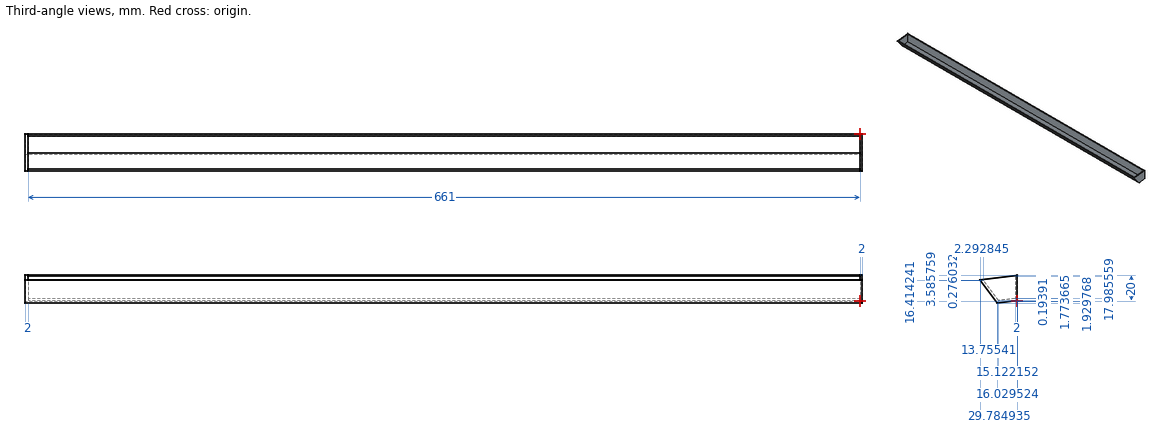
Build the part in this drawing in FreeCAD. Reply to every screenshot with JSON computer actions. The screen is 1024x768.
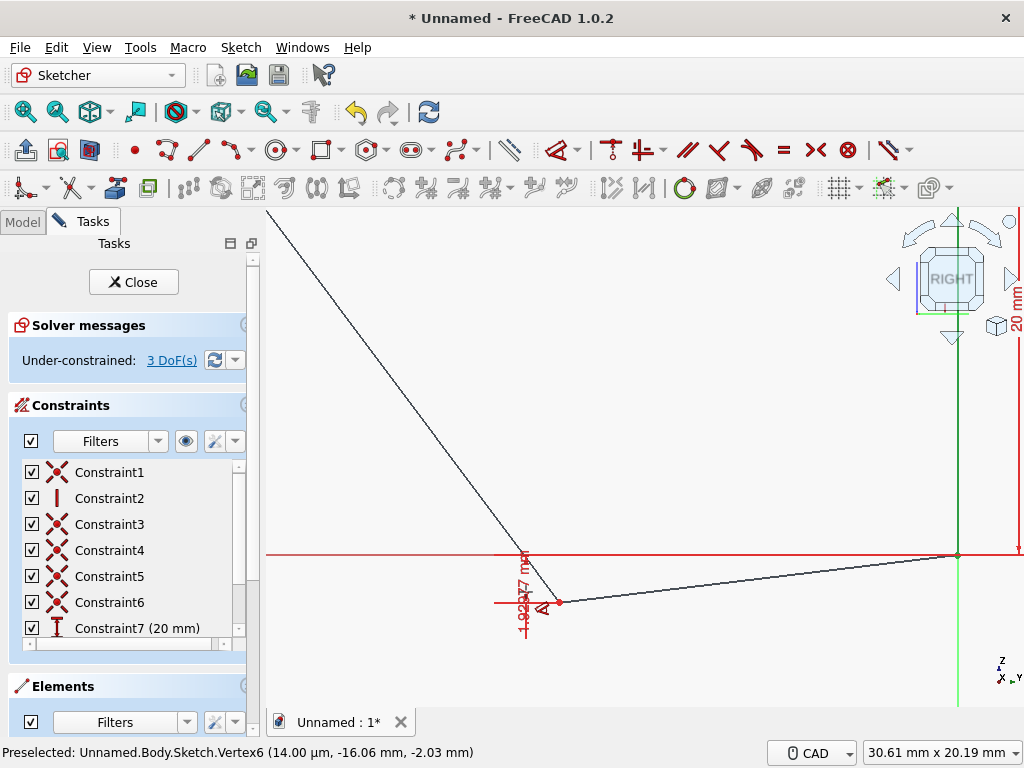
{"action": "scroll", "coordinate": [562, 610], "scroll_direction": "down", "scroll_amount": 3}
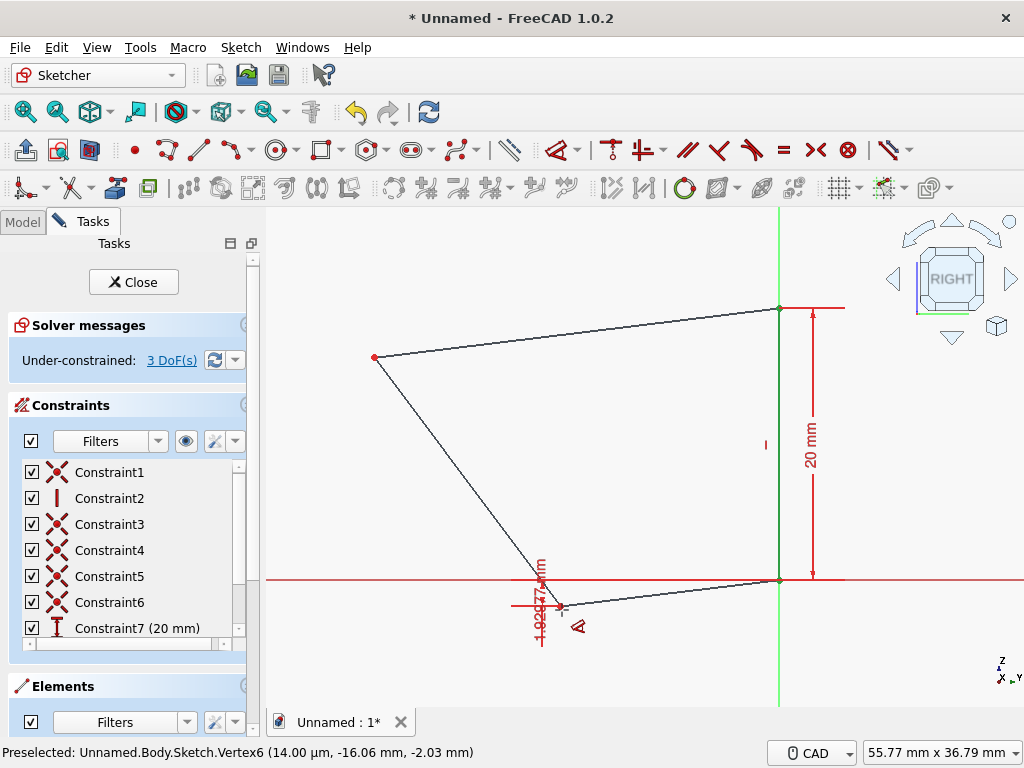
{"action": "left_click", "coordinate": [658, 323]}
{"action": "left_click", "coordinate": [813, 333]}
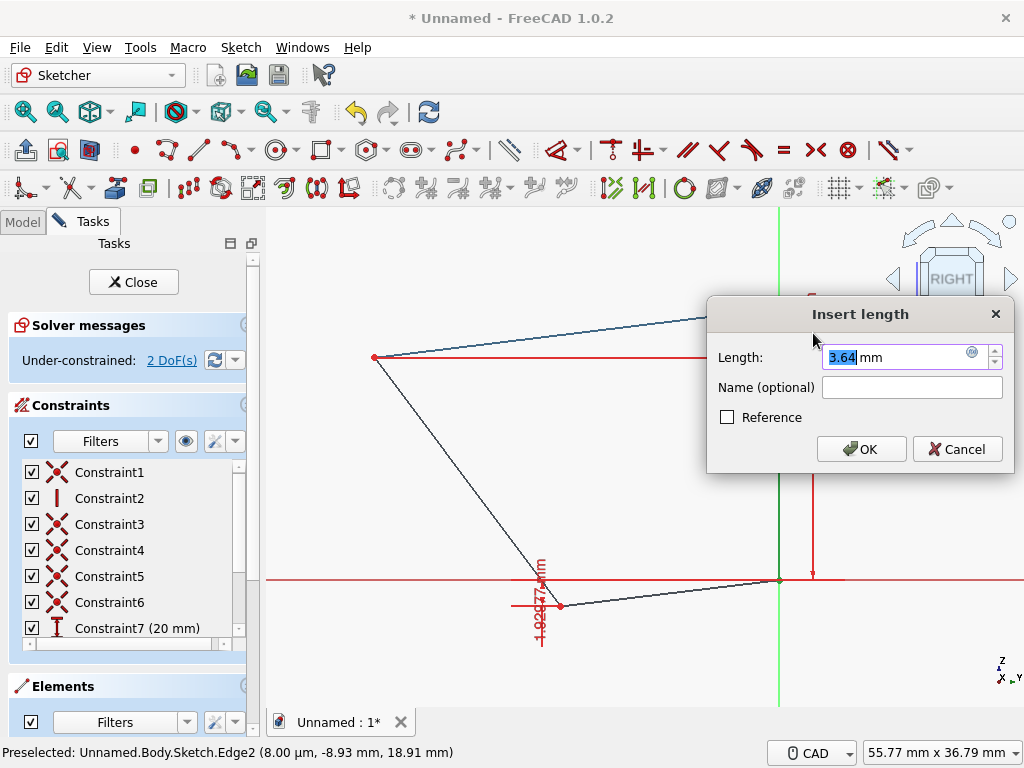
{"action": "type", "text": "3.585759"}
{"action": "key", "text": "Return"}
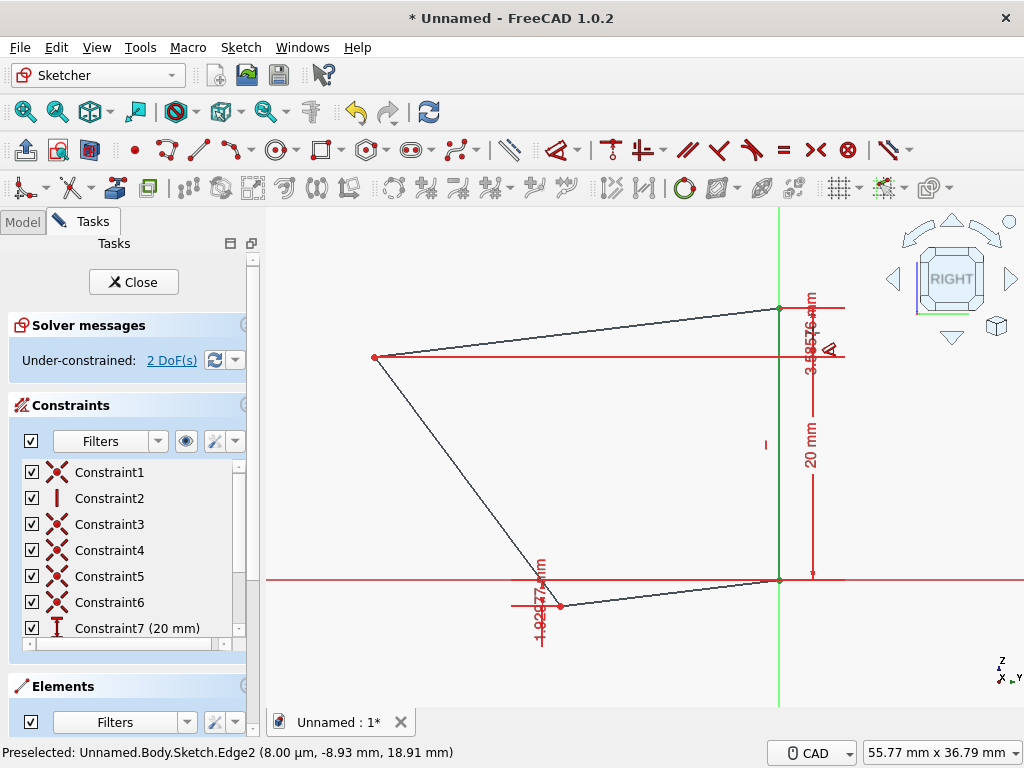
{"action": "left_click", "coordinate": [431, 432]}
{"action": "left_click", "coordinate": [468, 640]}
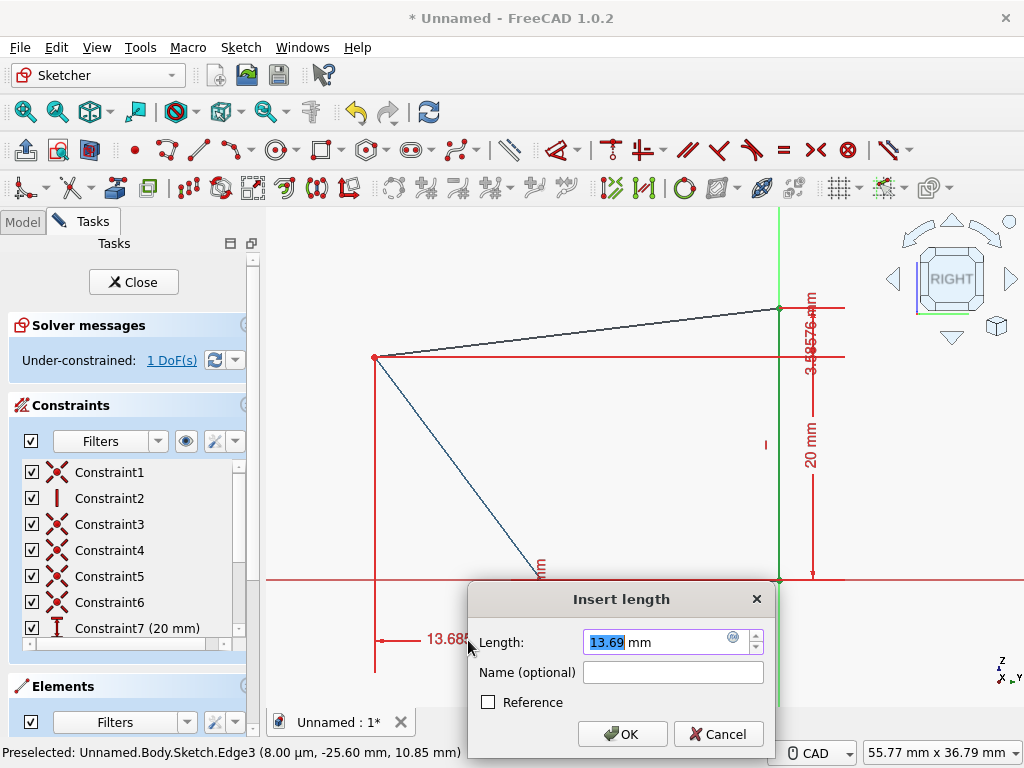
{"action": "type", "text": "13.75541"}
{"action": "key", "text": "Return"}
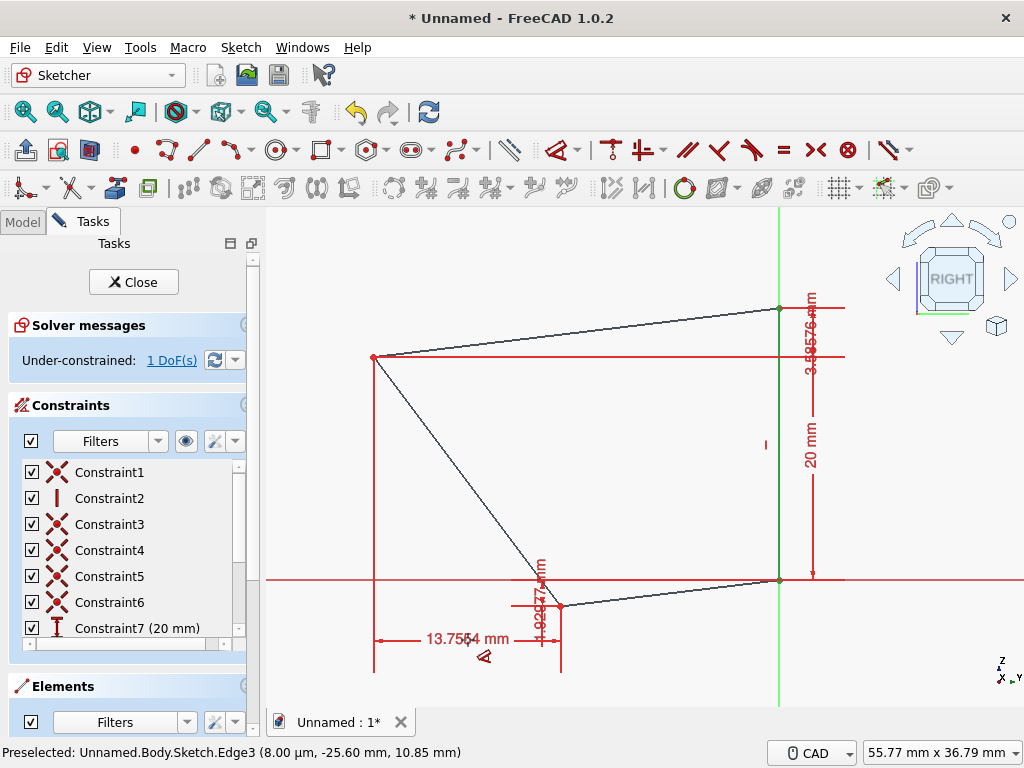
{"action": "left_click", "coordinate": [374, 357]}
{"action": "left_click", "coordinate": [670, 614]}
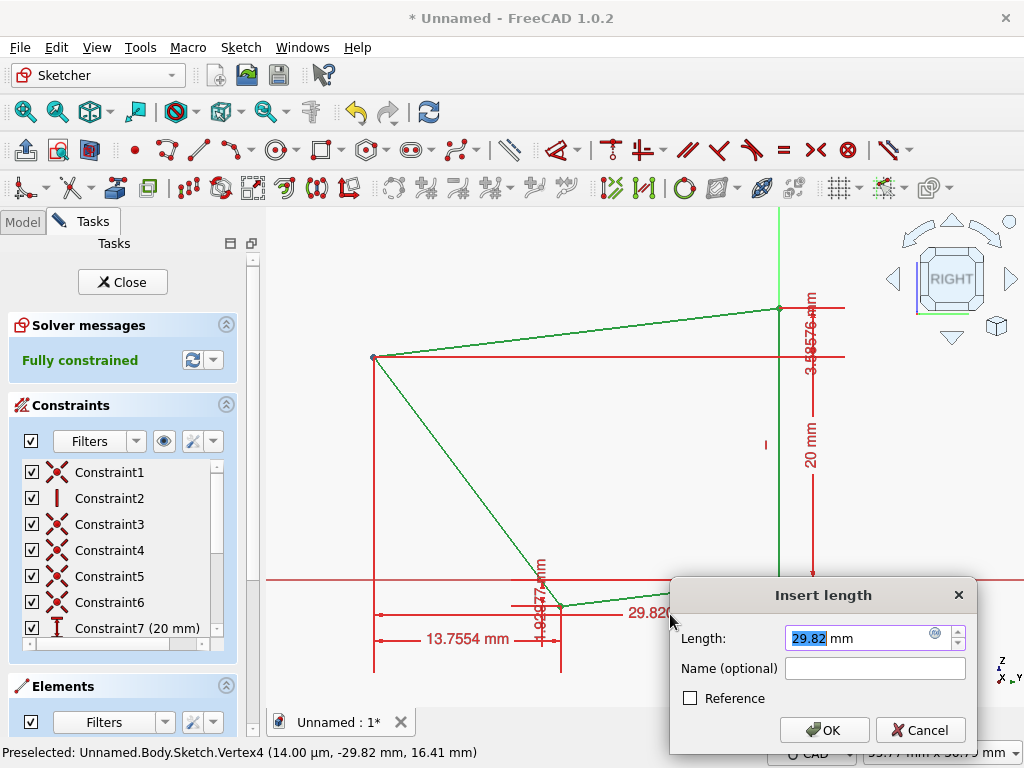
{"action": "type", "text": "29.784935"}
{"action": "key", "text": "Return"}
{"action": "key", "text": "Escape"}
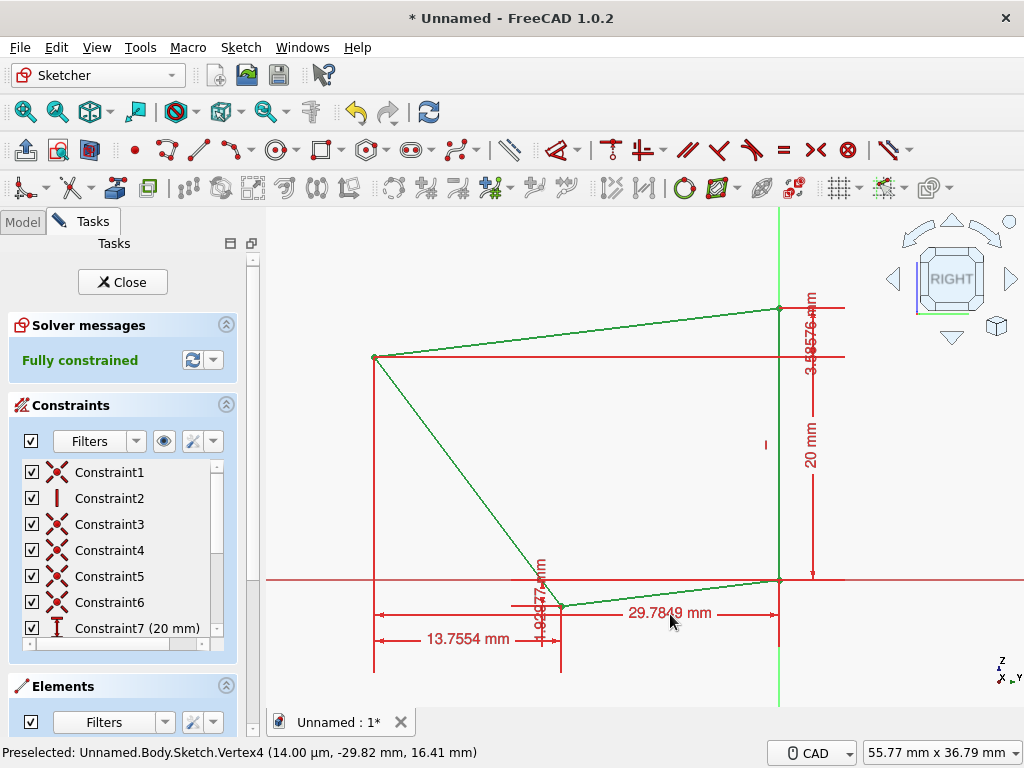
{"action": "left_click", "coordinate": [123, 282]}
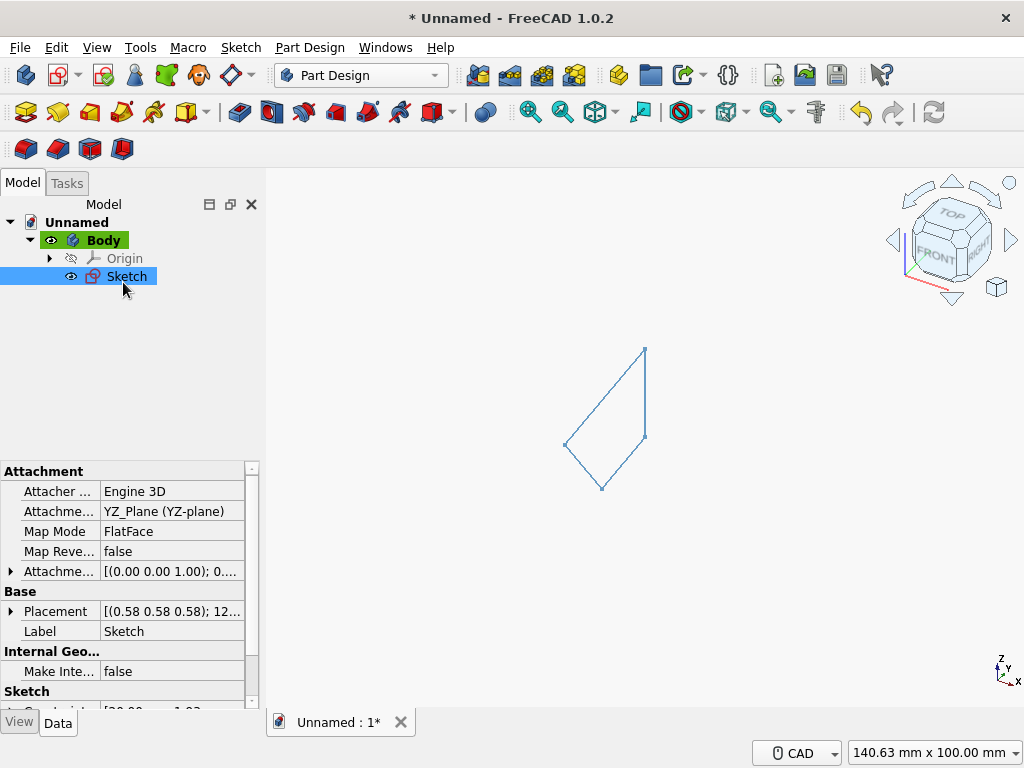
{"action": "left_click", "coordinate": [26, 112]}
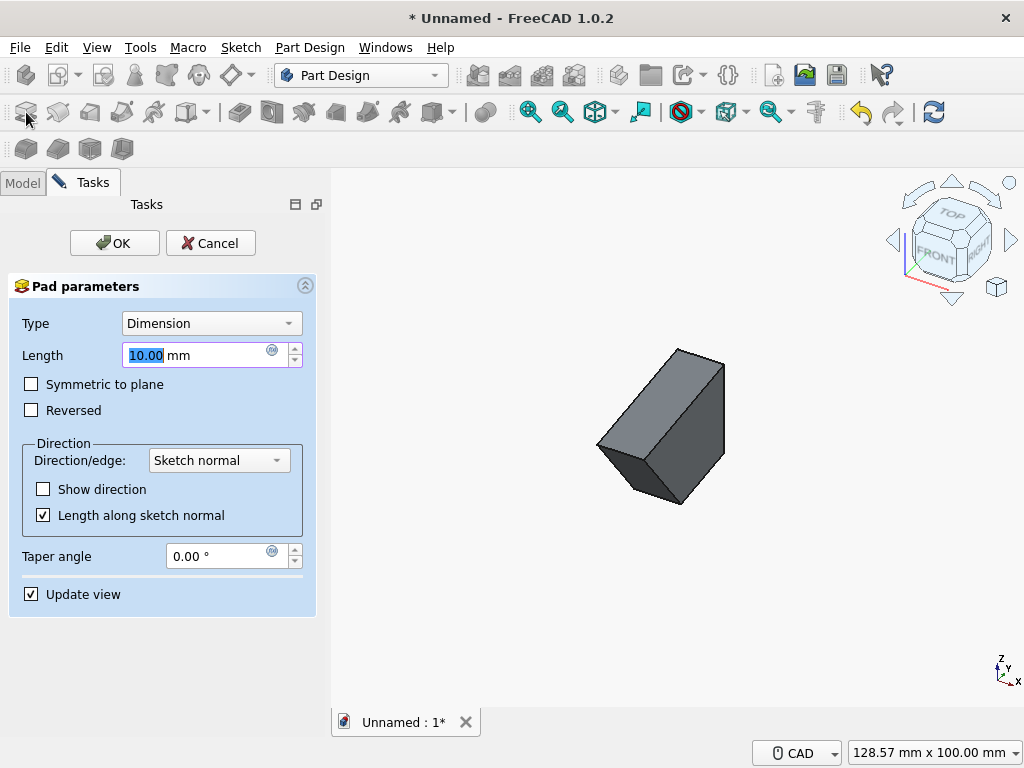
{"action": "type", "text": "2"}
{"action": "key", "text": "Tab"}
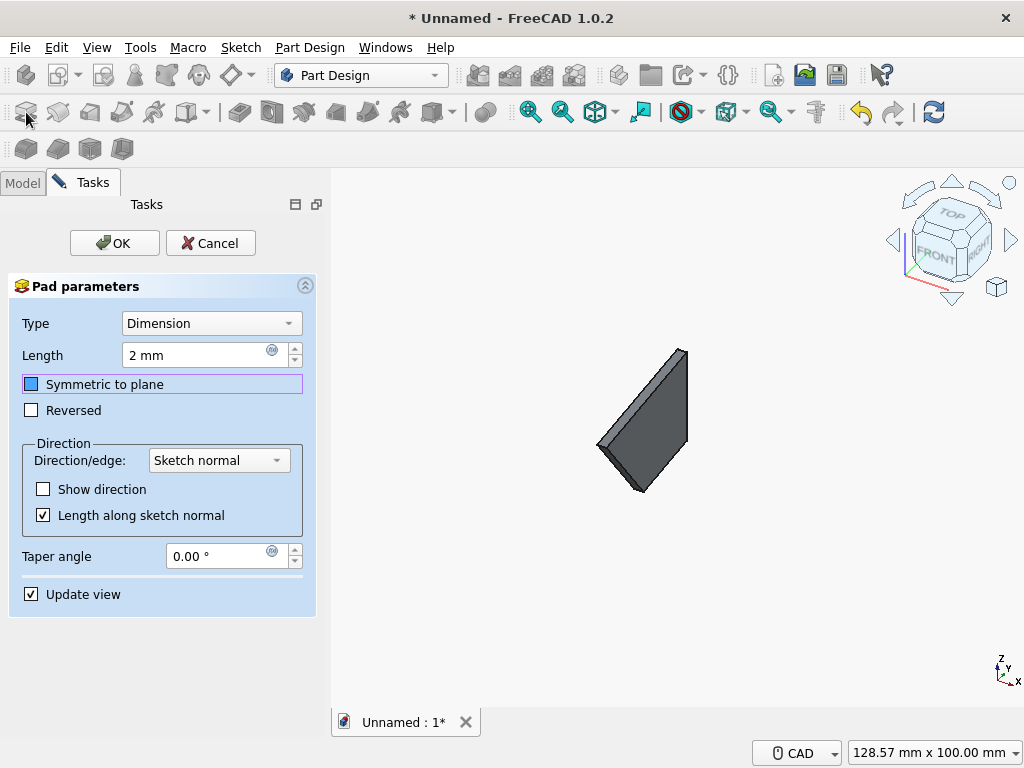
{"action": "left_click", "coordinate": [115, 243]}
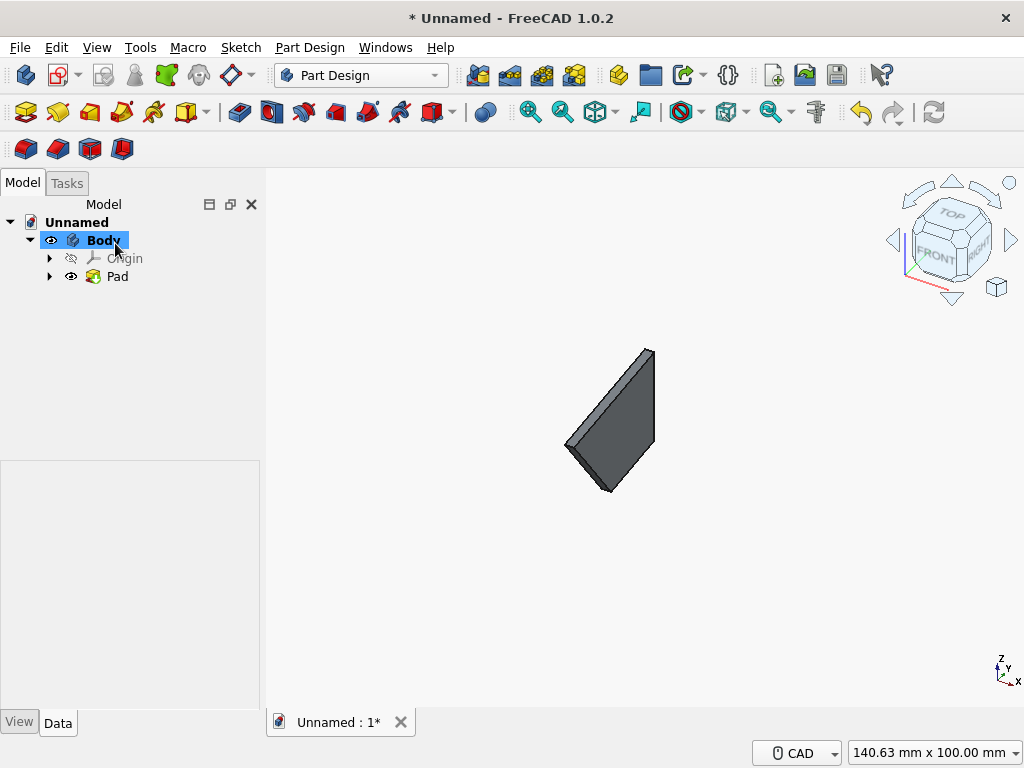
{"action": "key", "text": "v f"}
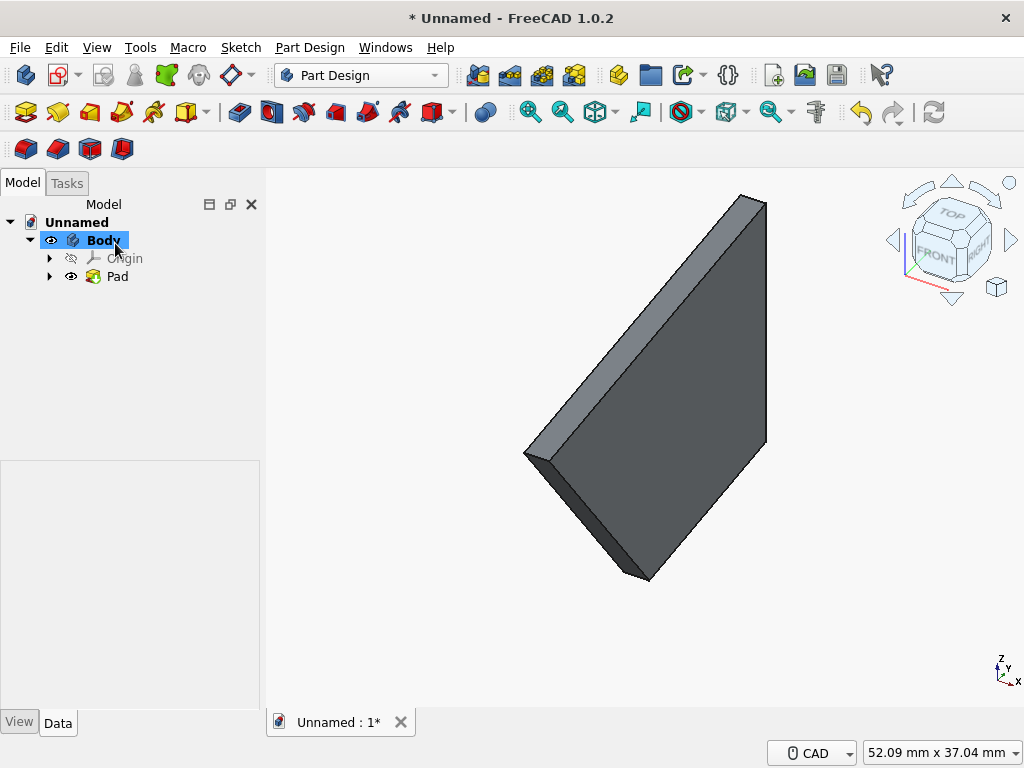
{"action": "key", "text": "6"}